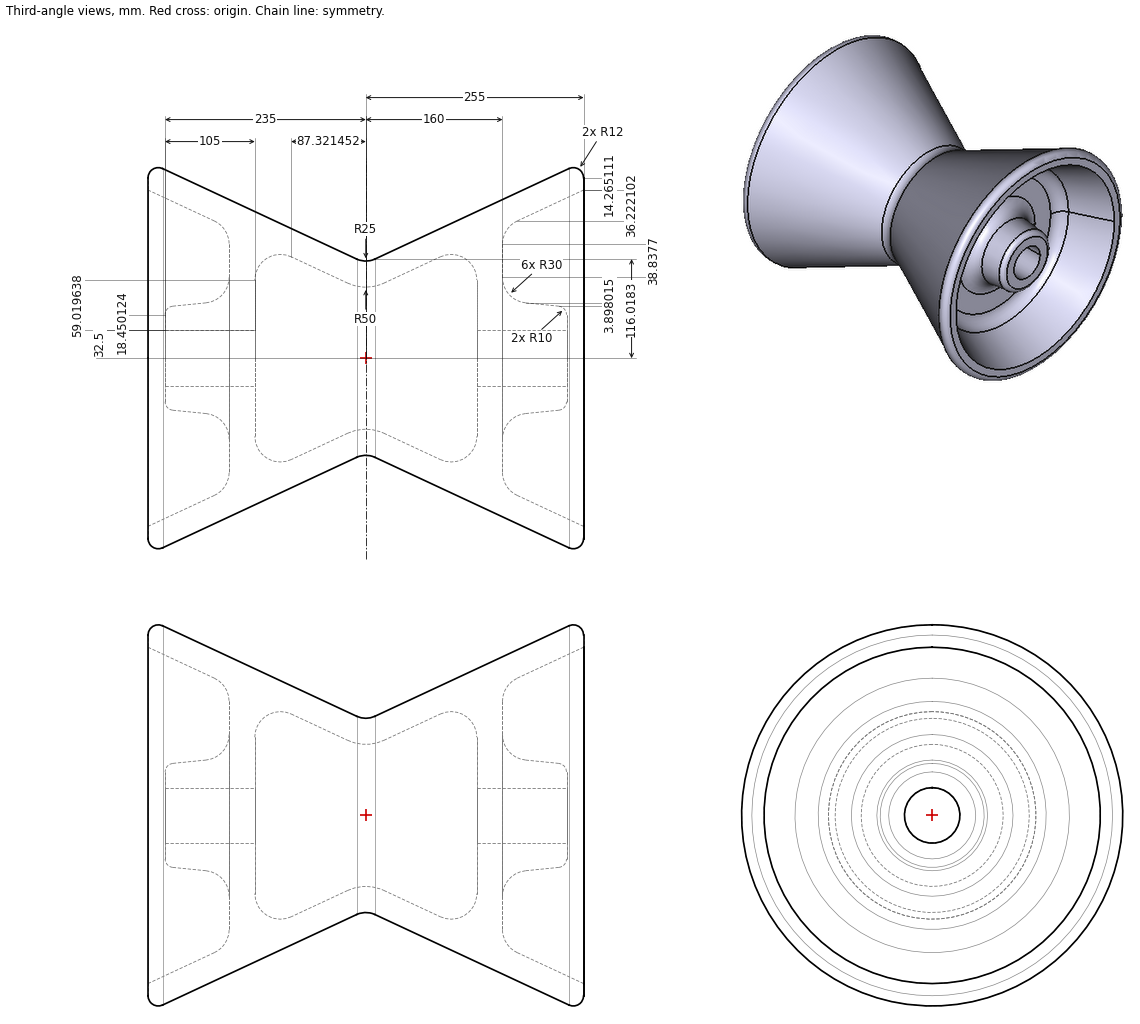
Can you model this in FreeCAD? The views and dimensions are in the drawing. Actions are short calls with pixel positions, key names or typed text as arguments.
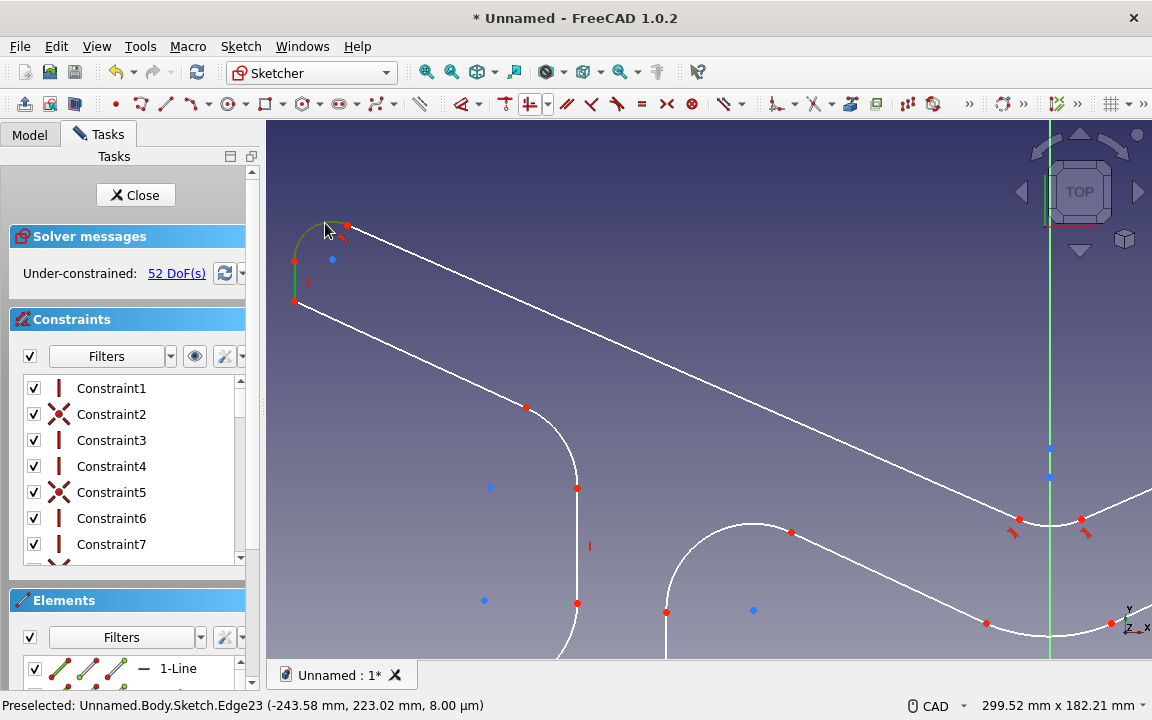
click(617, 104)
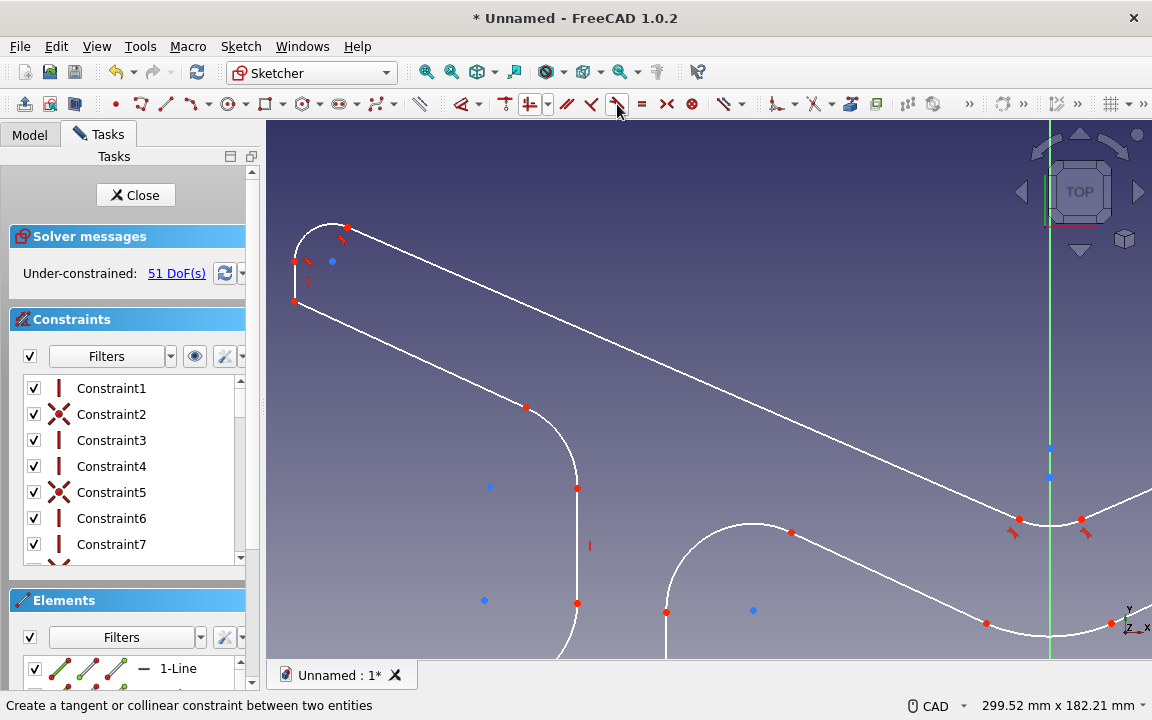
click(364, 333)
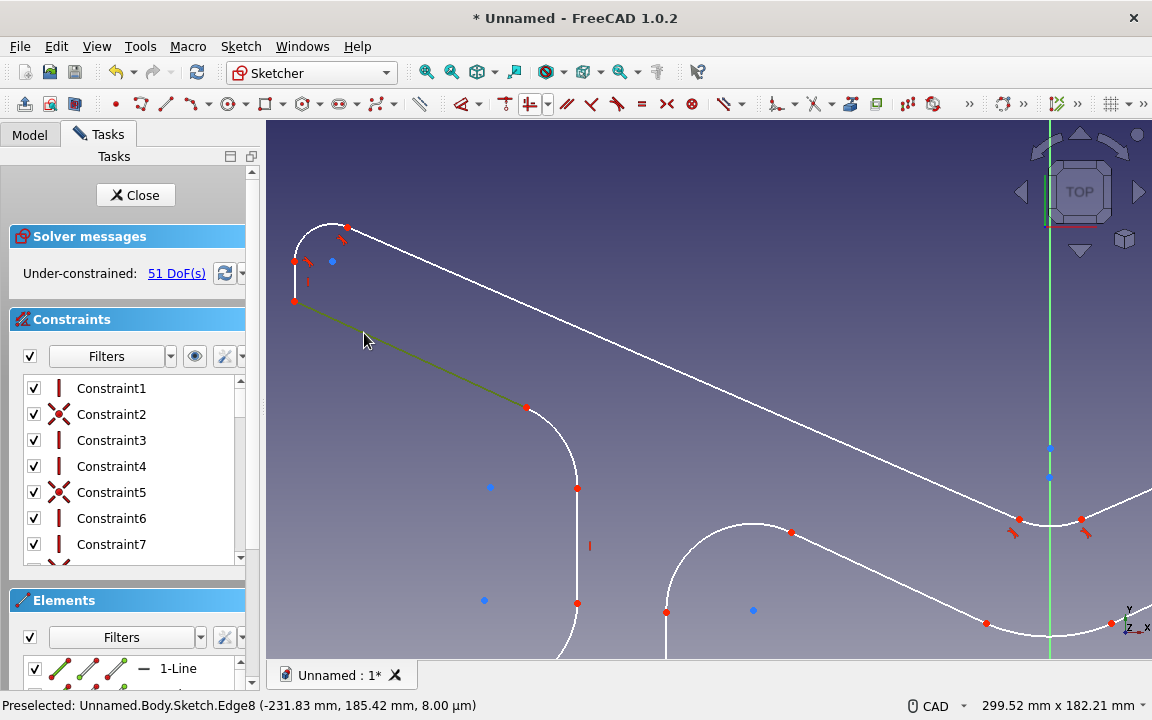
click(573, 458)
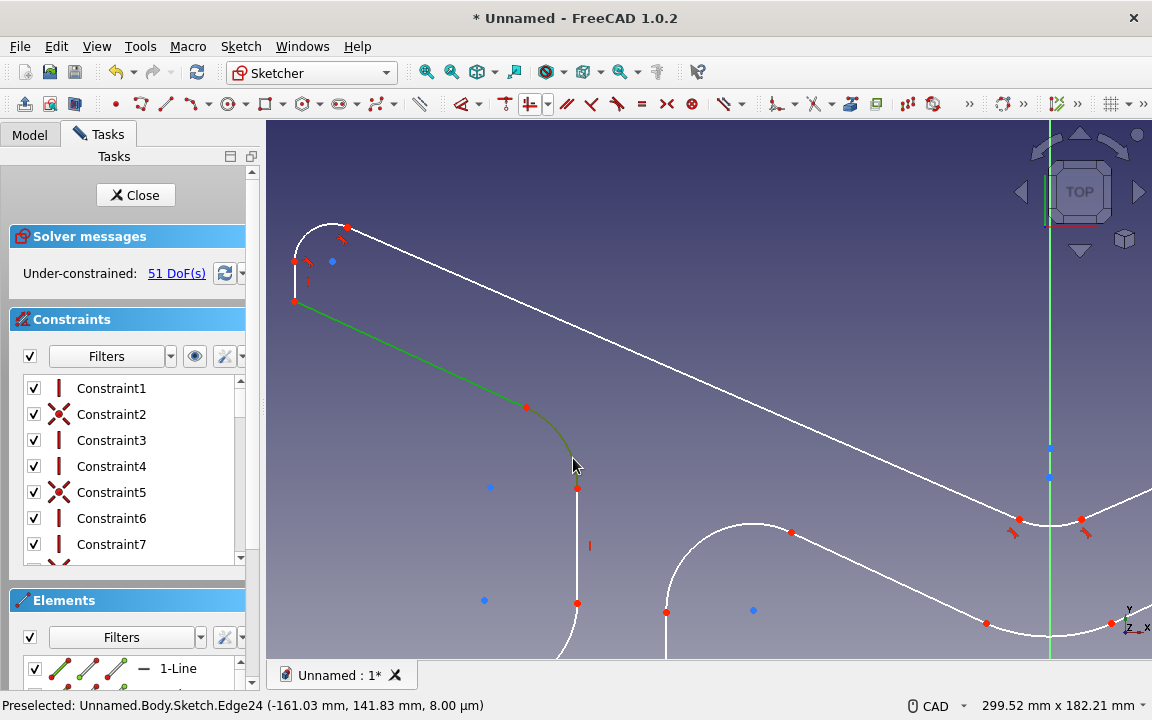
click(617, 104)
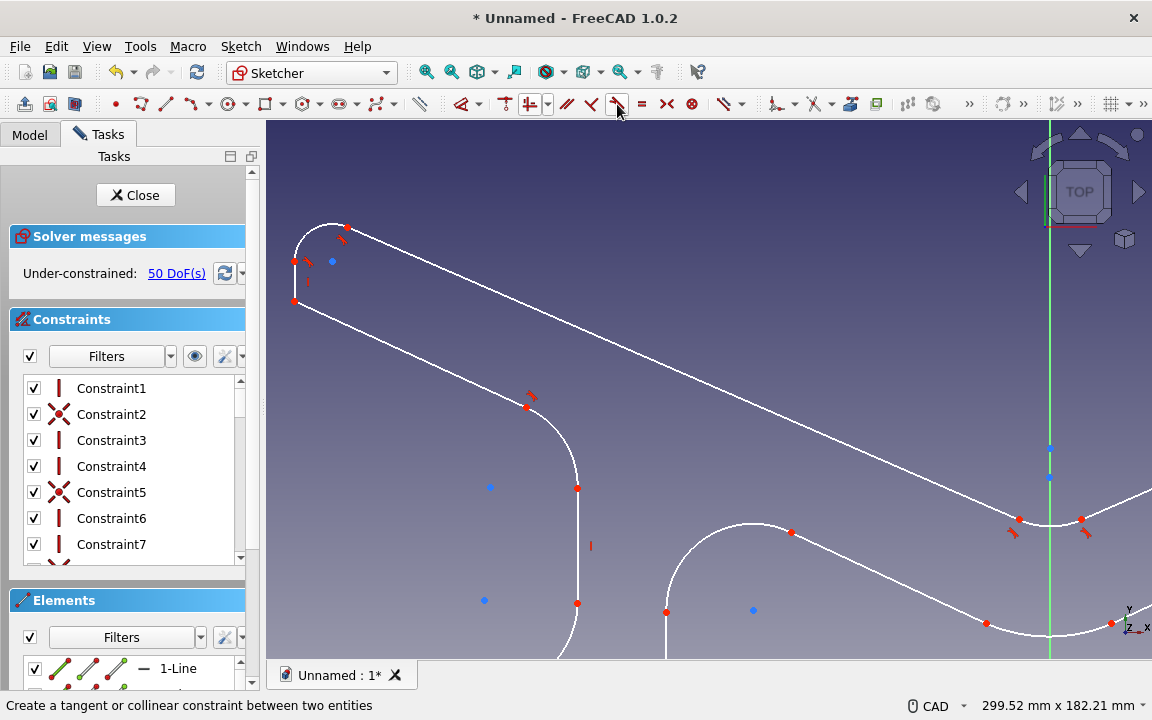
click(578, 523)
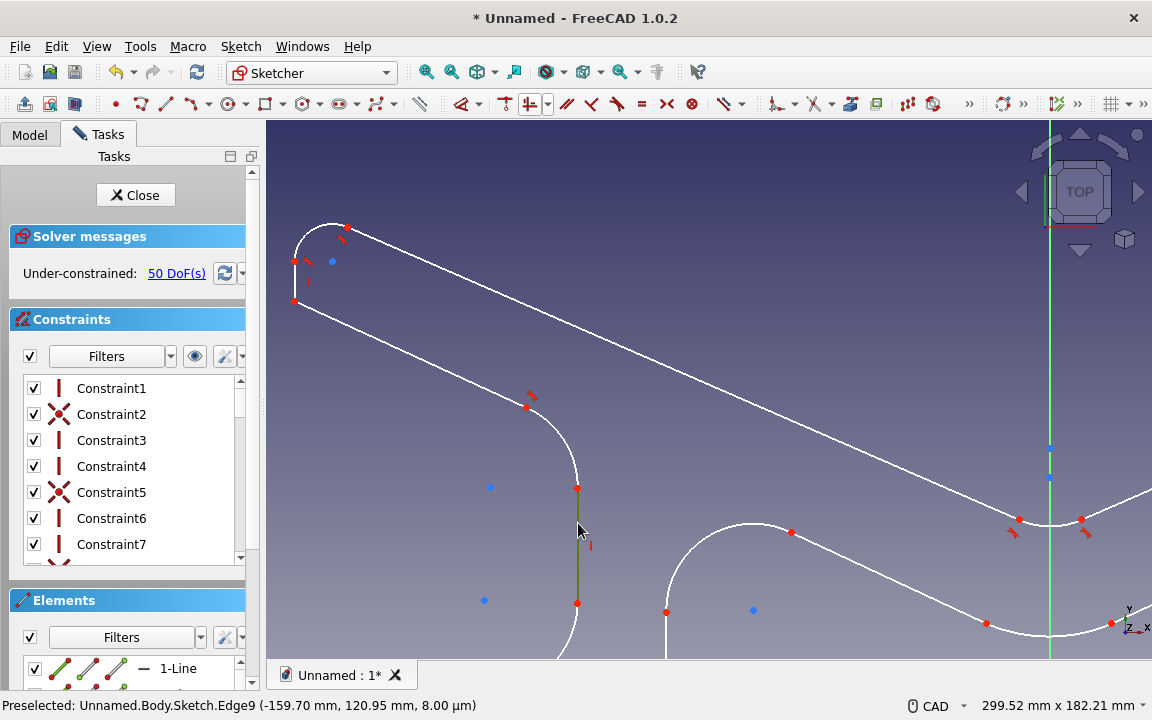
click(573, 459)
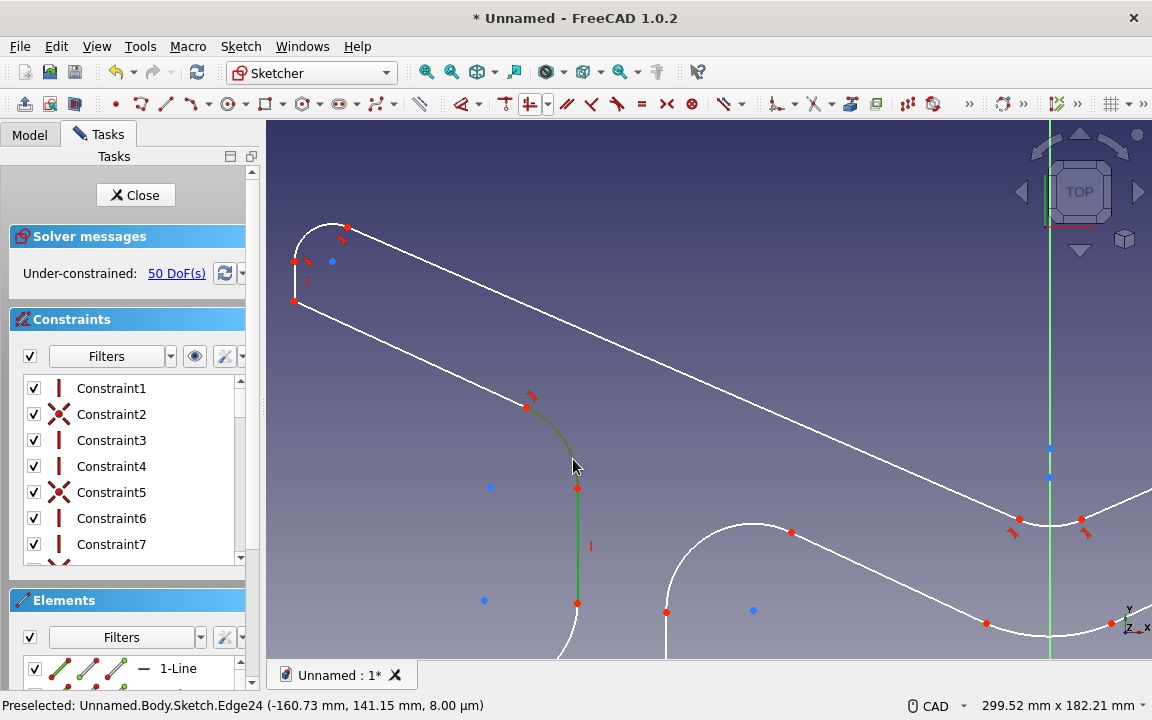
click(617, 104)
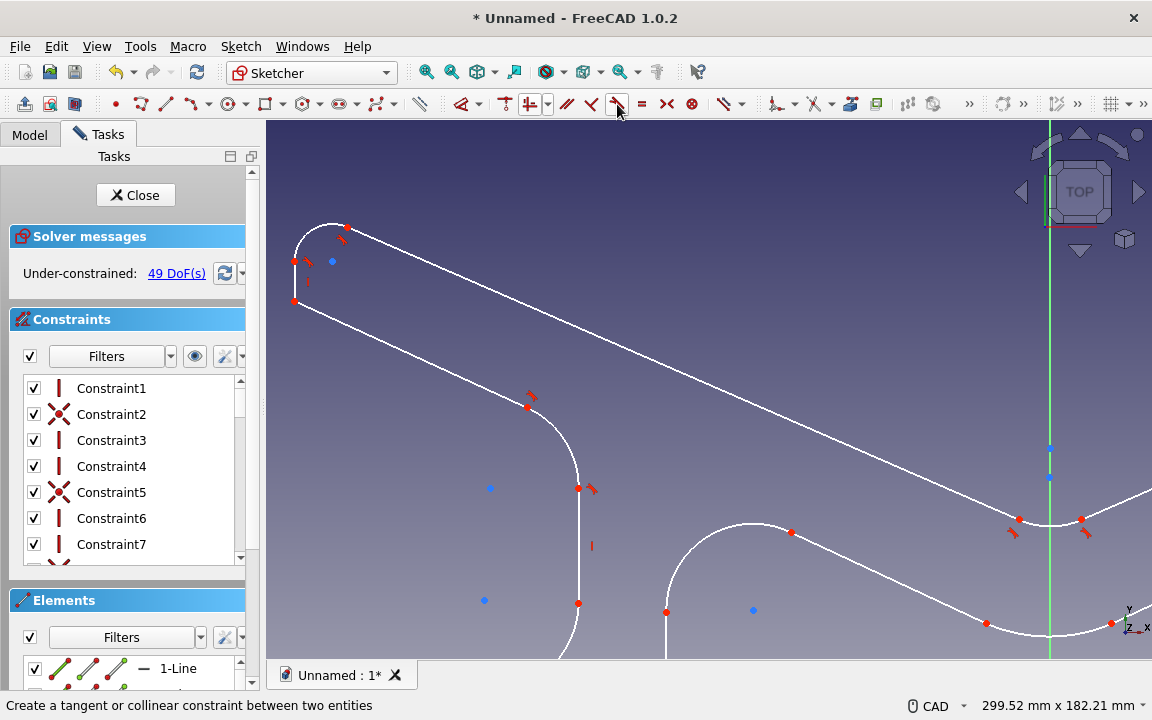
click(579, 523)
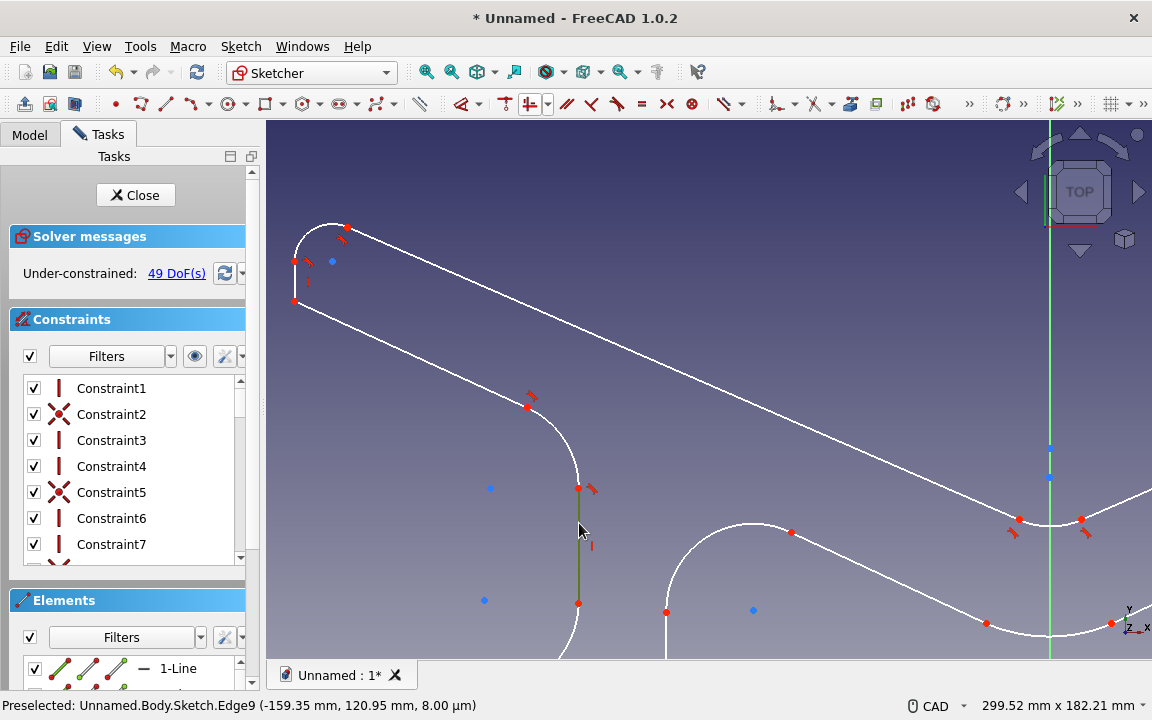
click(574, 630)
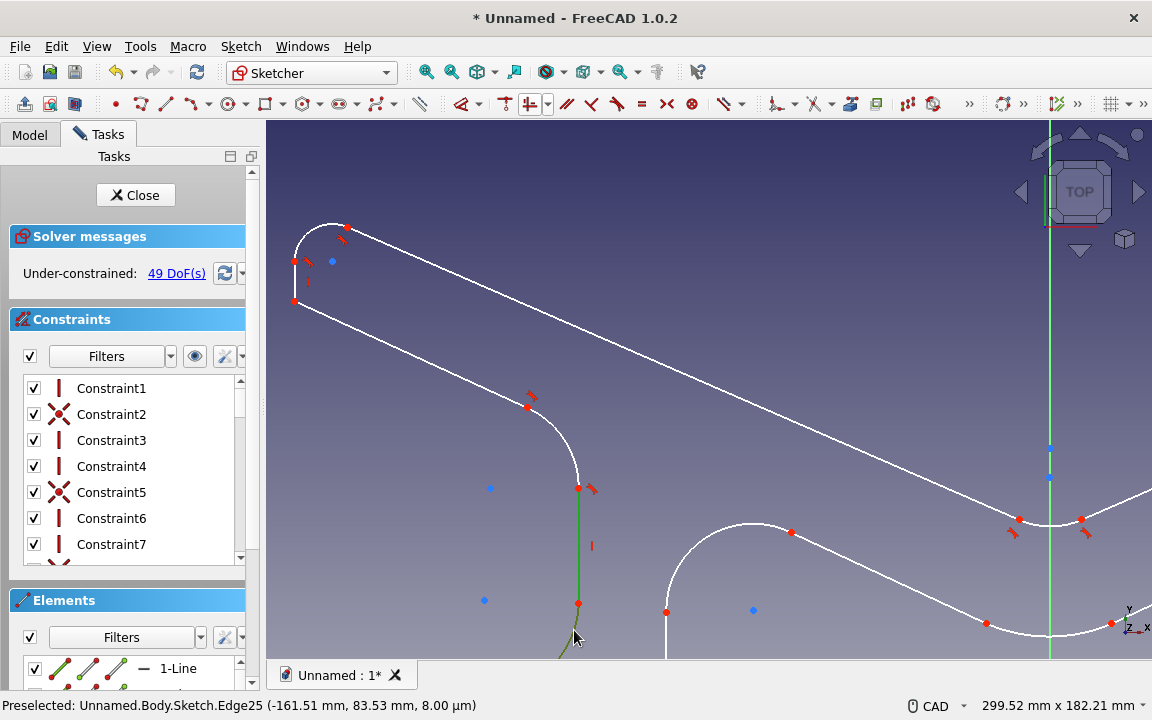
click(617, 104)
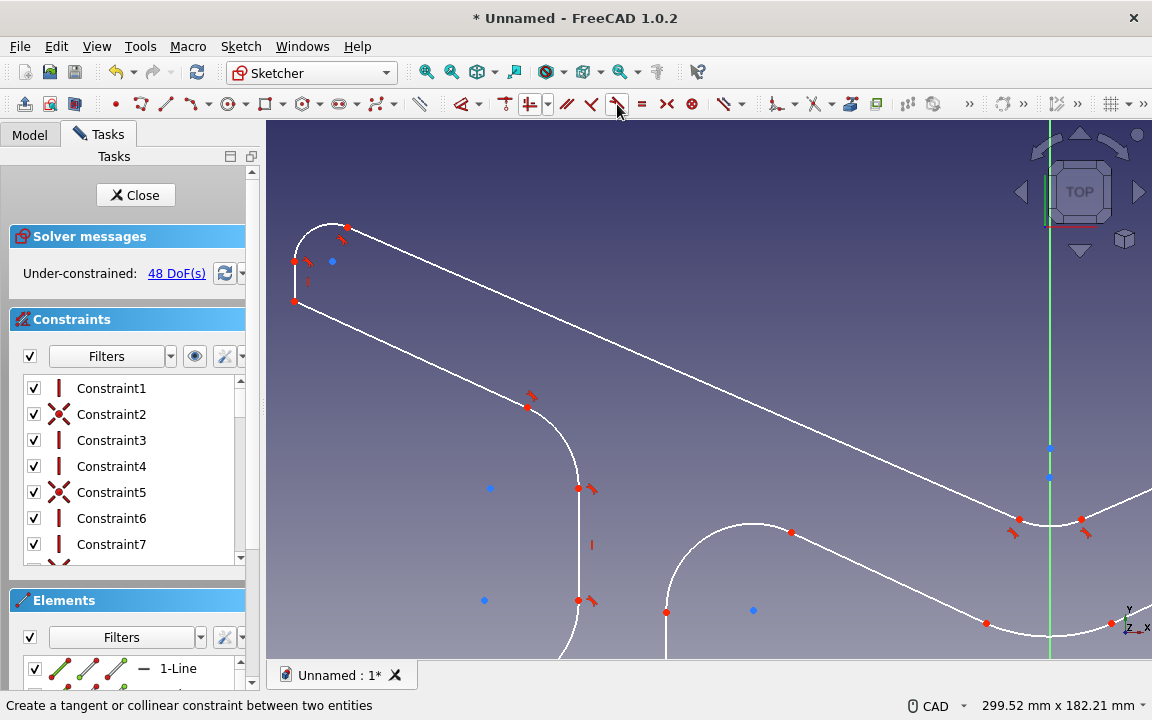
scroll(464, 319, down, 6)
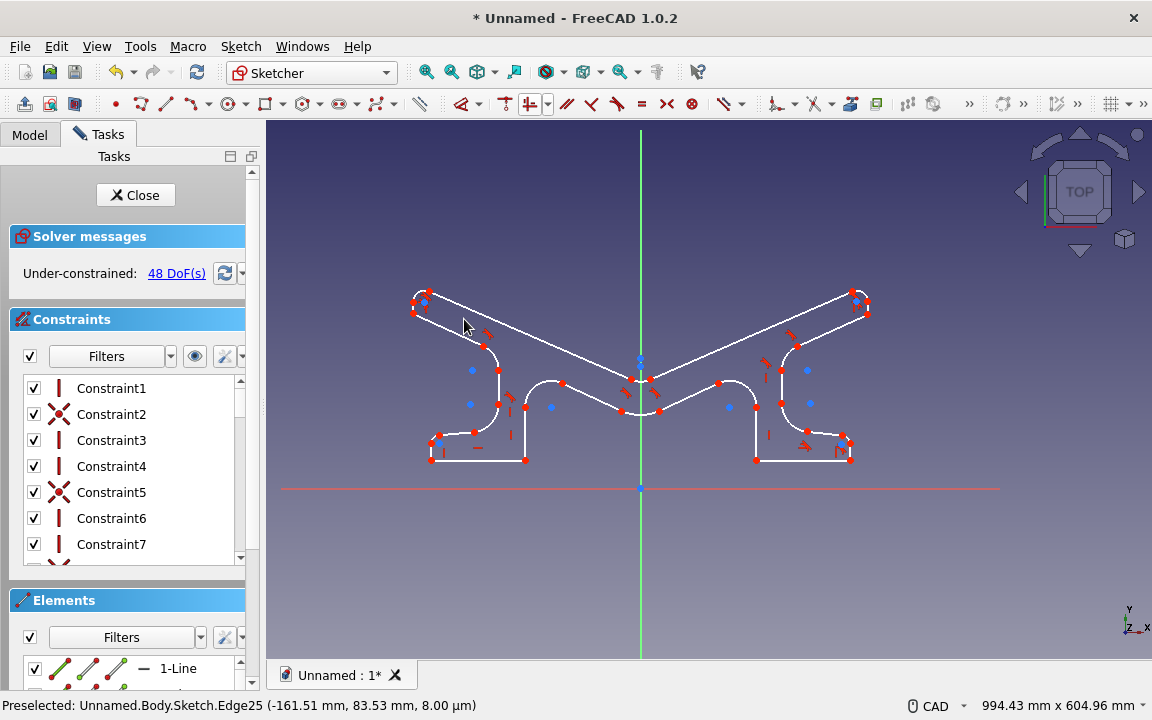
scroll(464, 433, up, 2)